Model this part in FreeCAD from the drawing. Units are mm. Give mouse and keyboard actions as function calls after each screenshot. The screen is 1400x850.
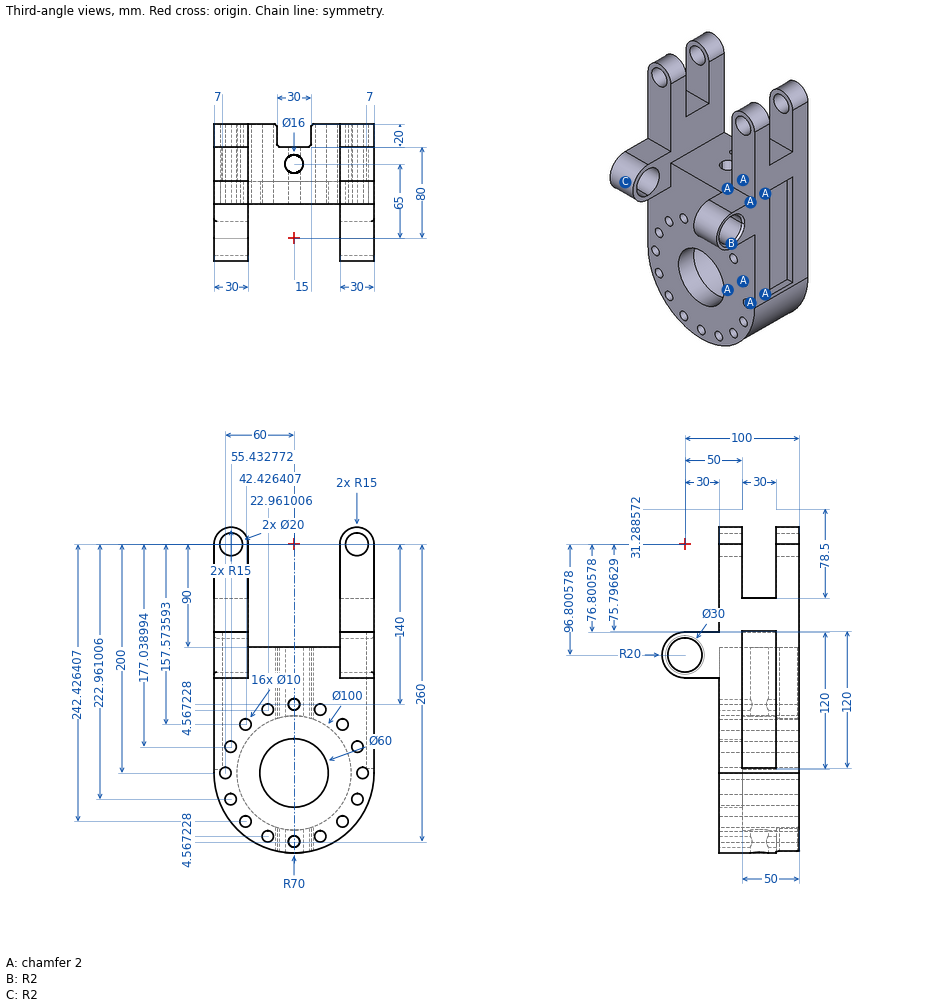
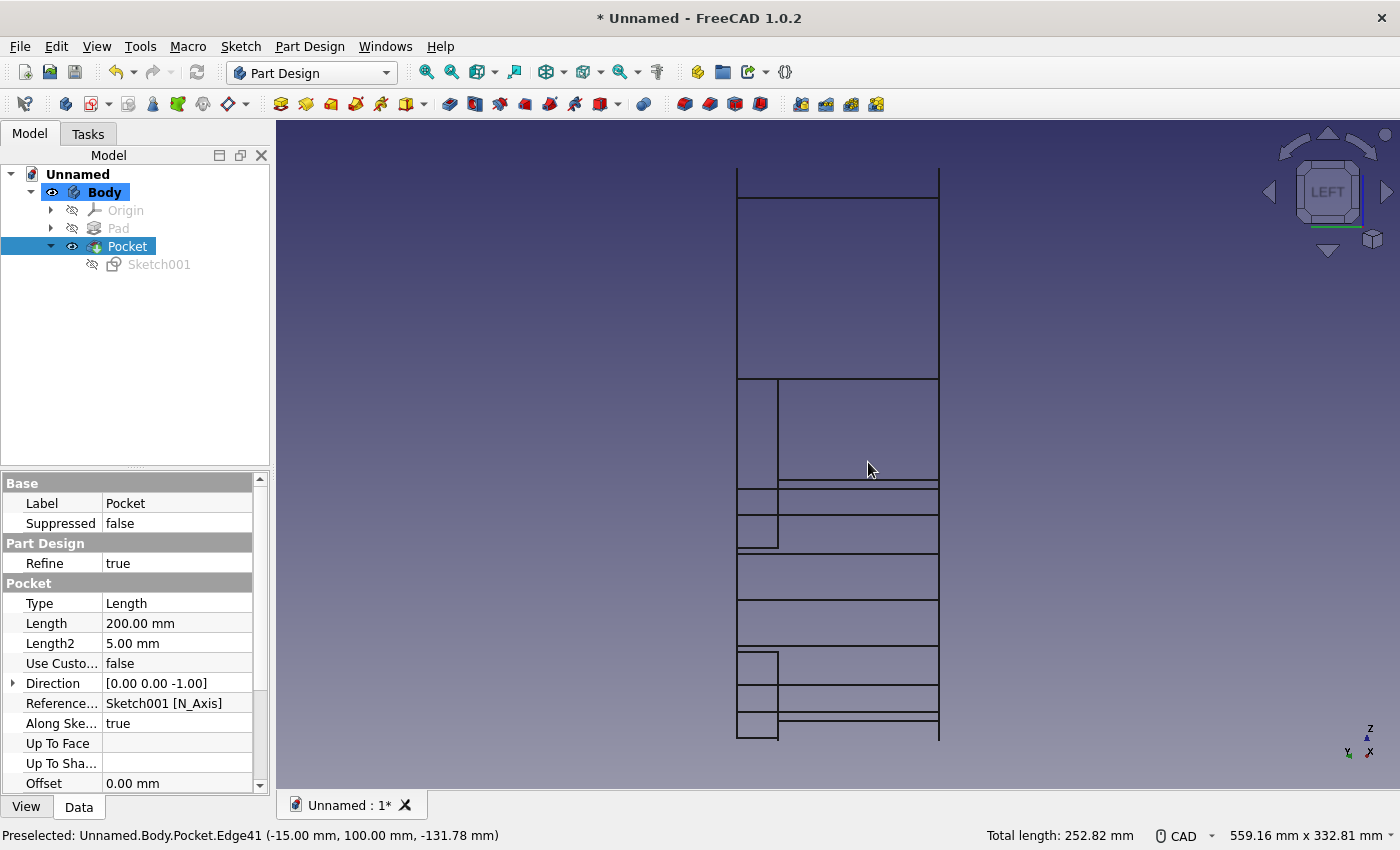
key(0)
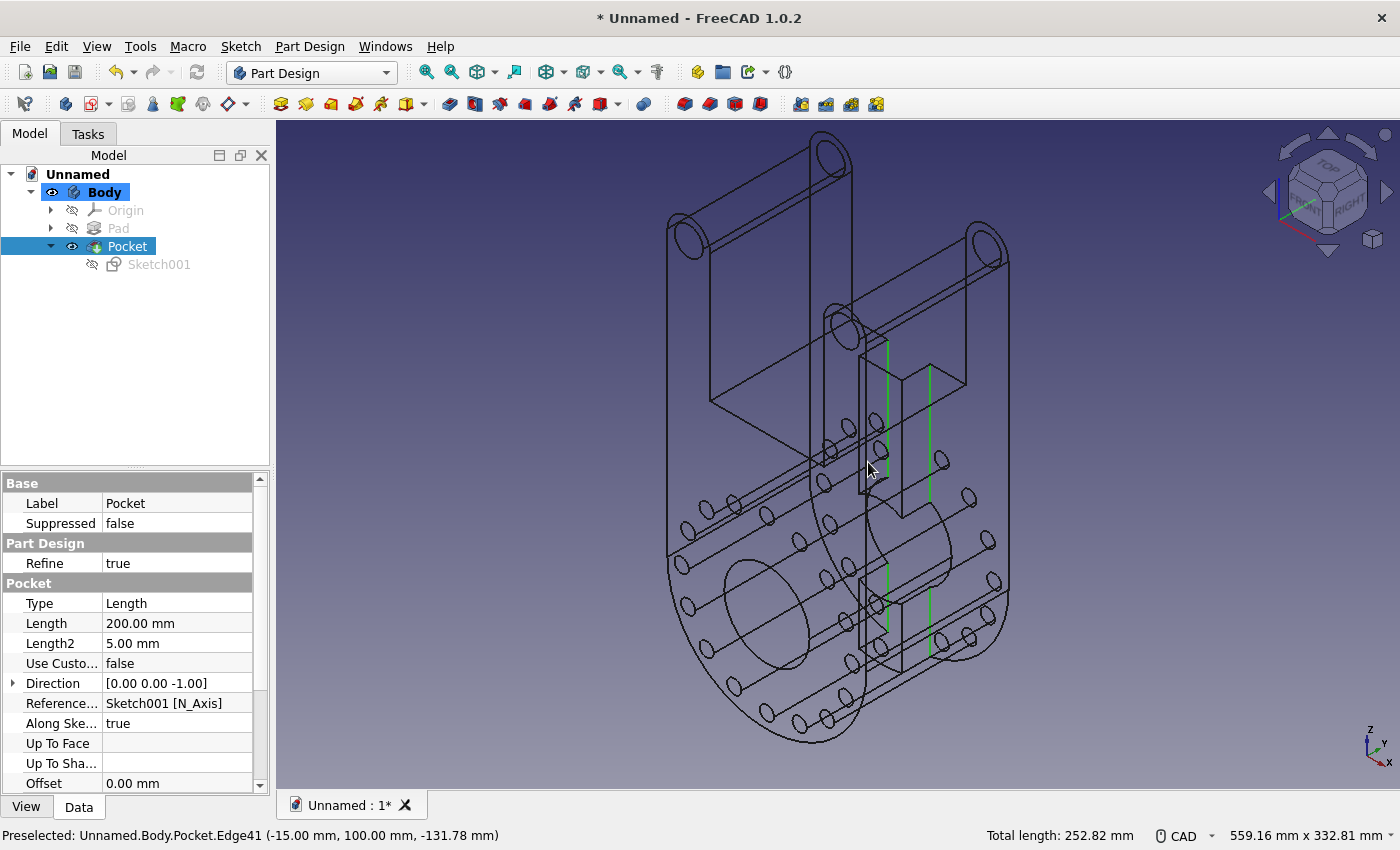
click(859, 599, ctrl)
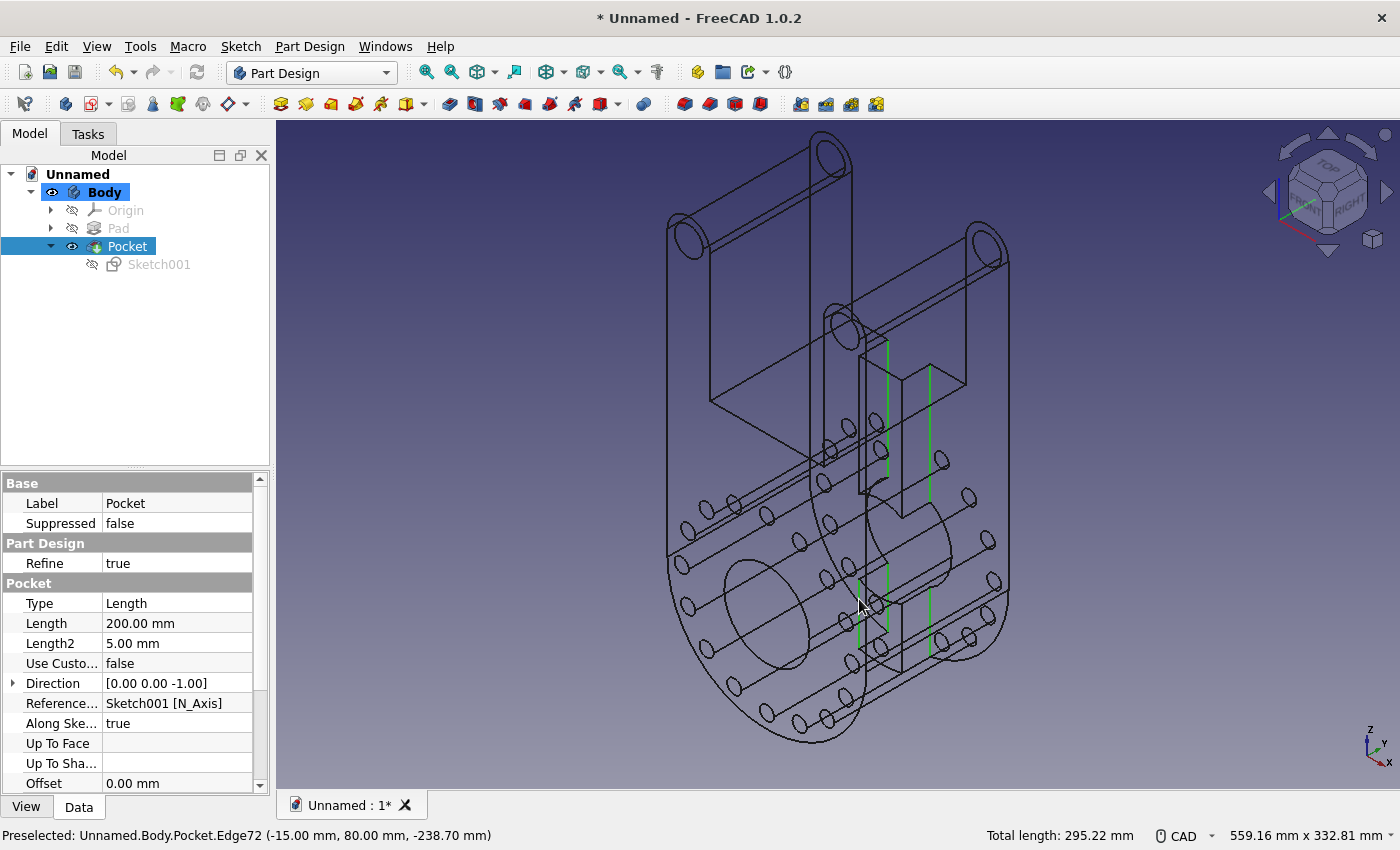
click(902, 631, ctrl)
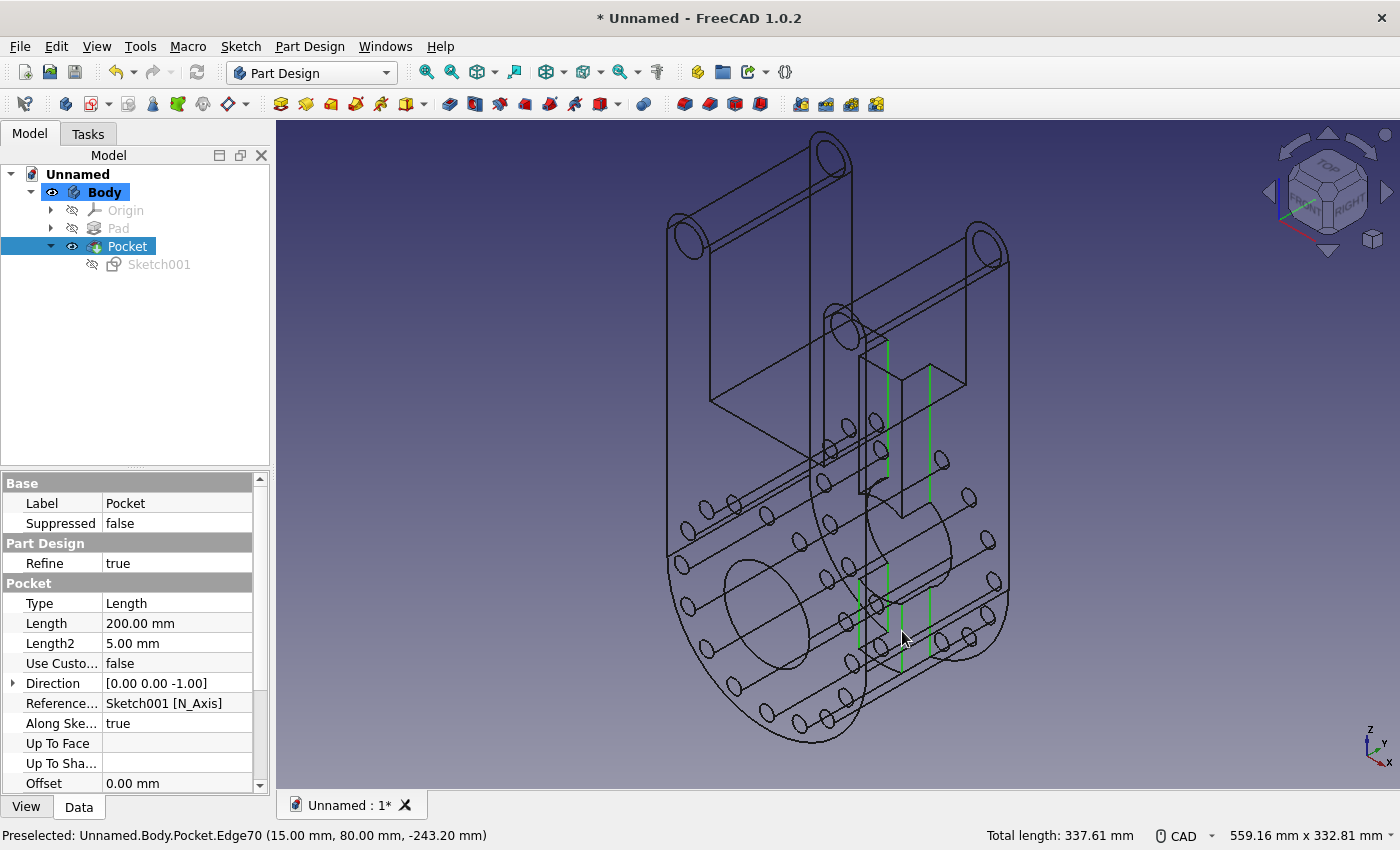
click(902, 449, ctrl)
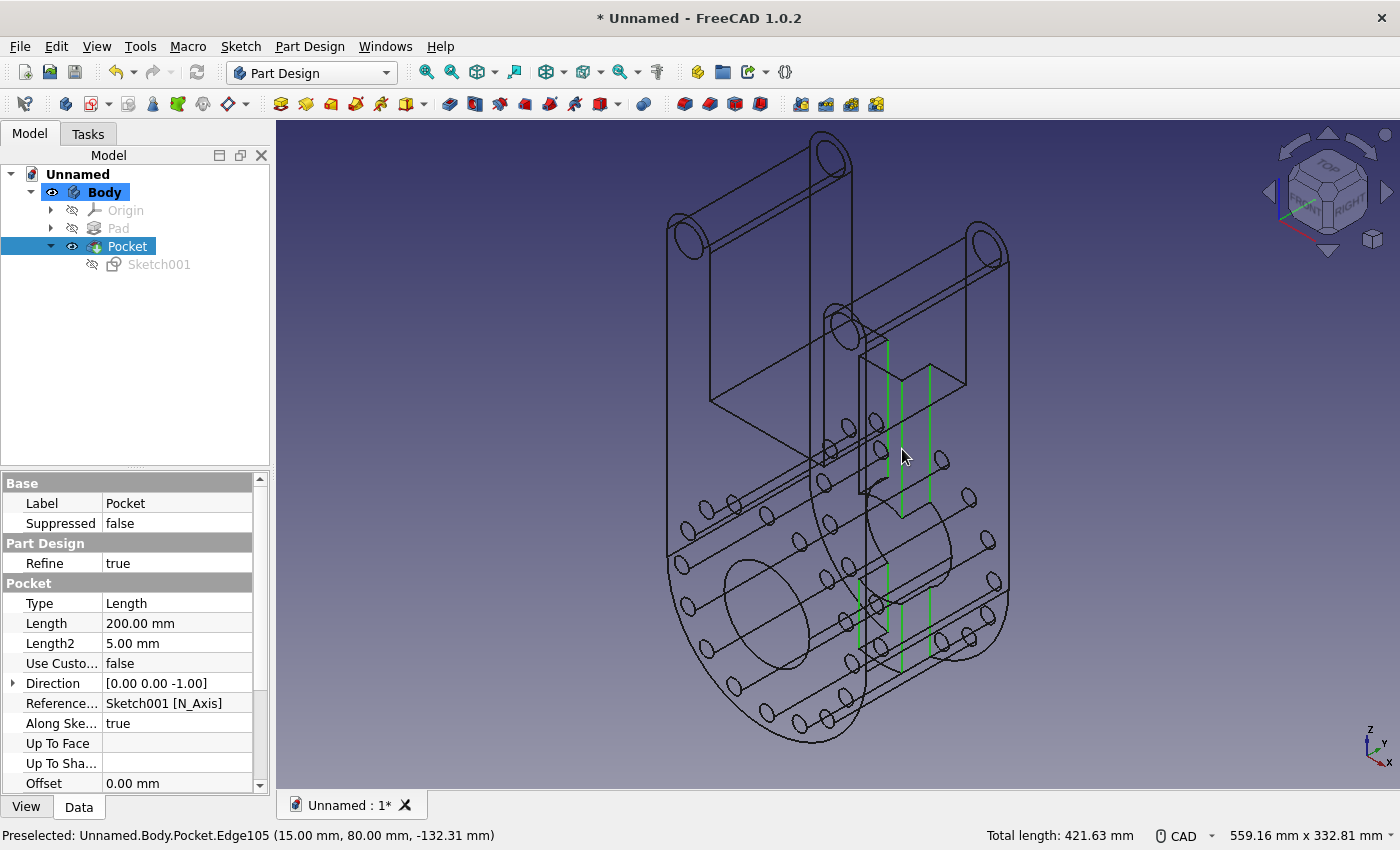
click(859, 424, ctrl)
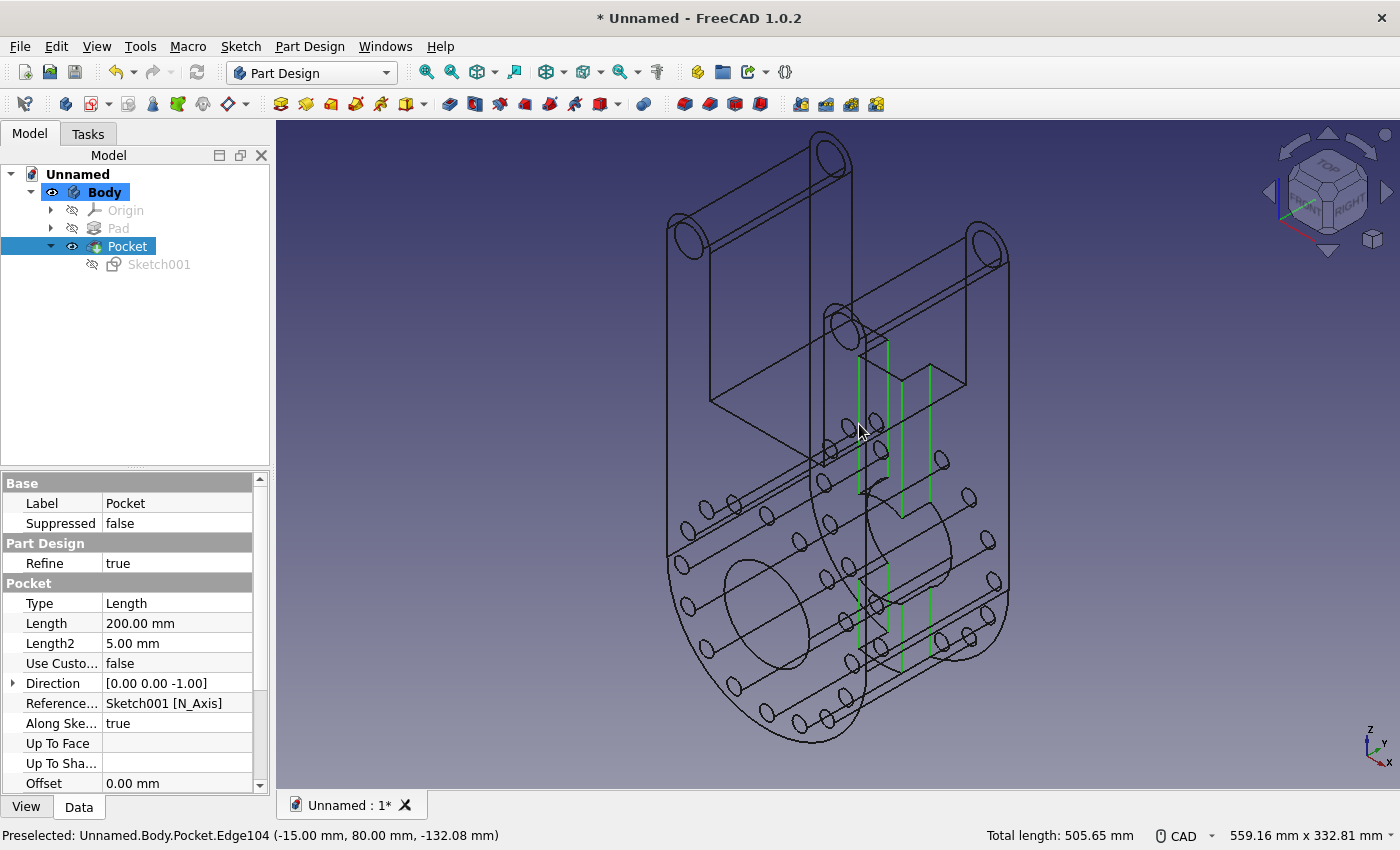
key(v)
key(1)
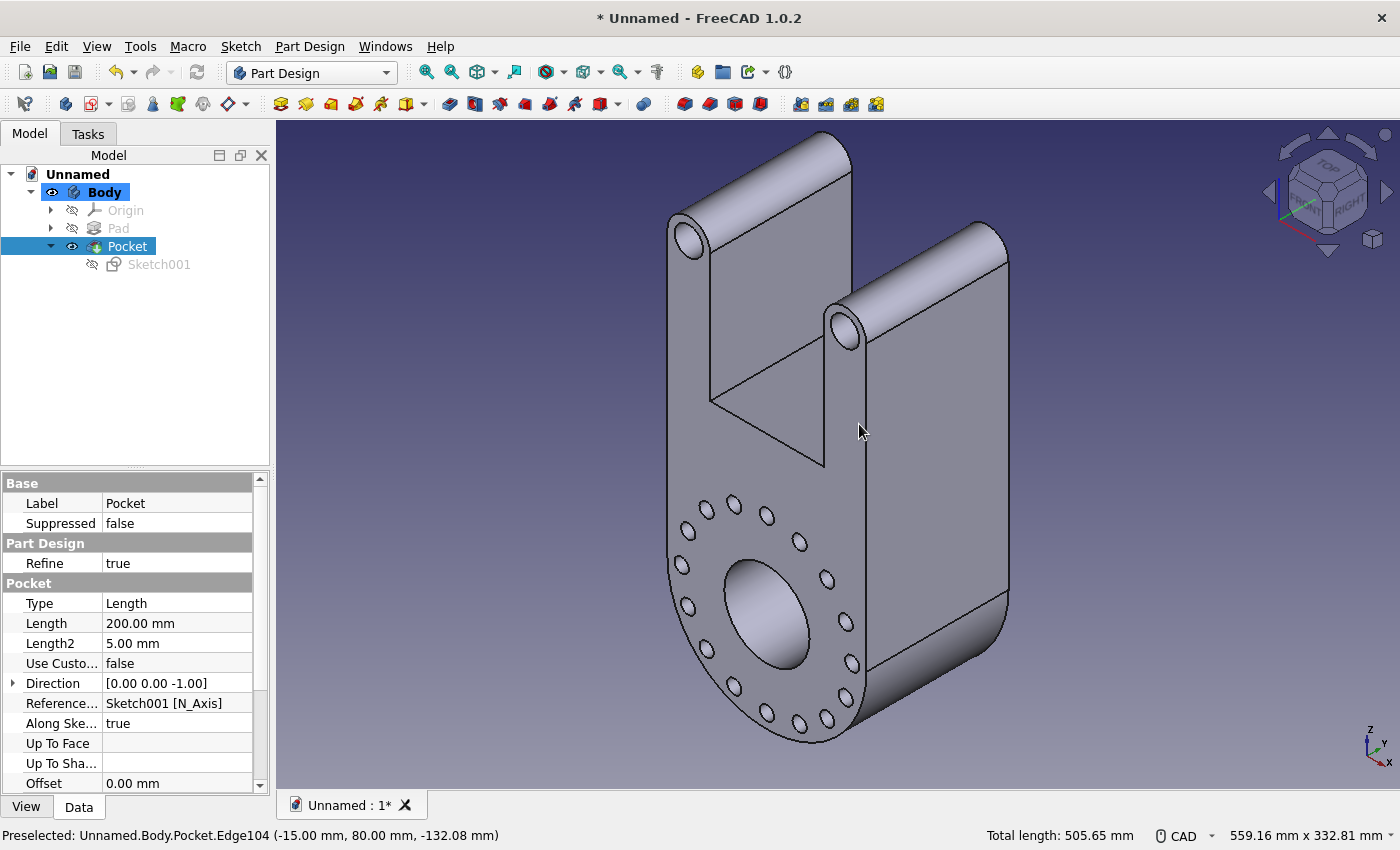
click(710, 104)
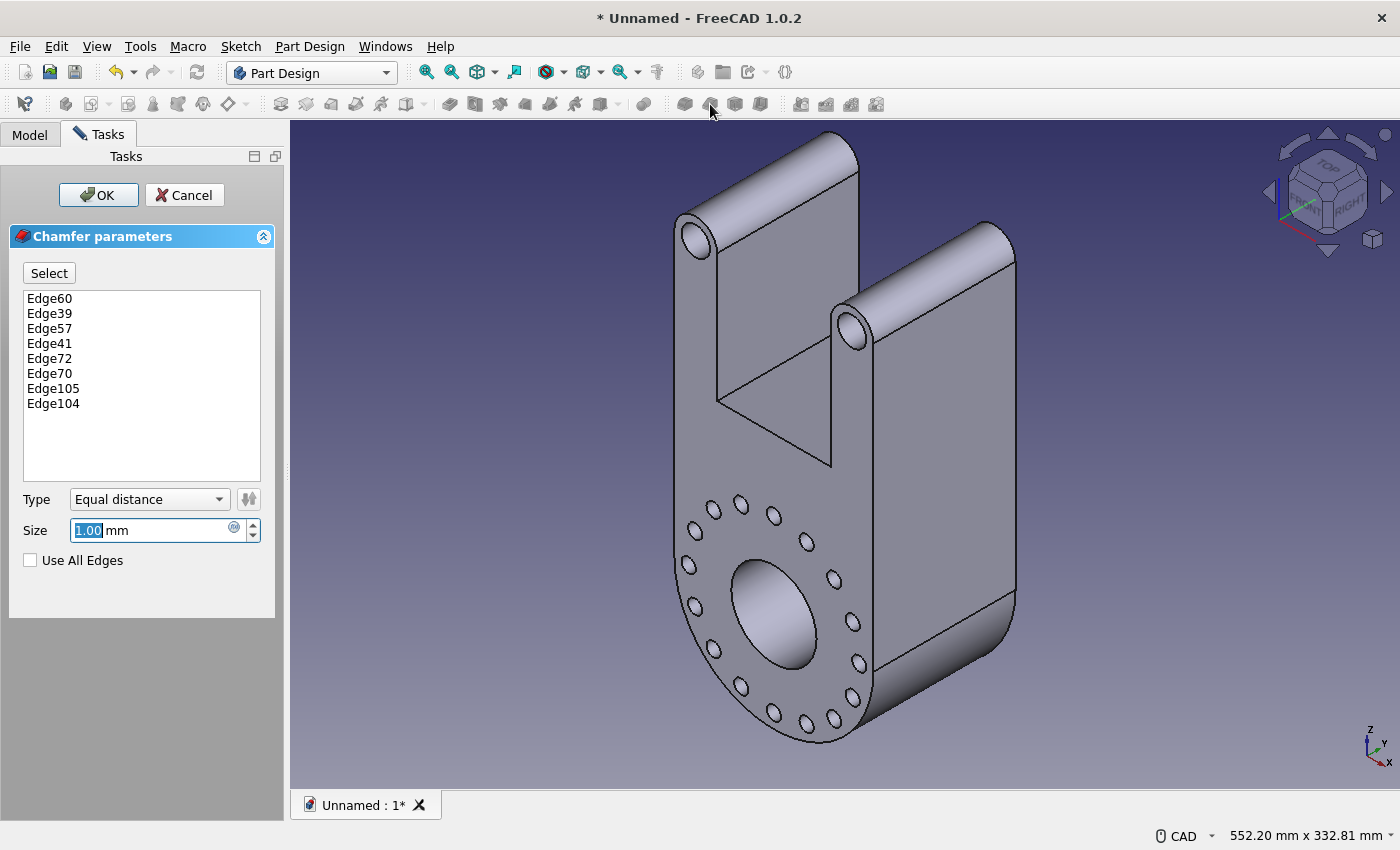
text(2)
key(Tab)